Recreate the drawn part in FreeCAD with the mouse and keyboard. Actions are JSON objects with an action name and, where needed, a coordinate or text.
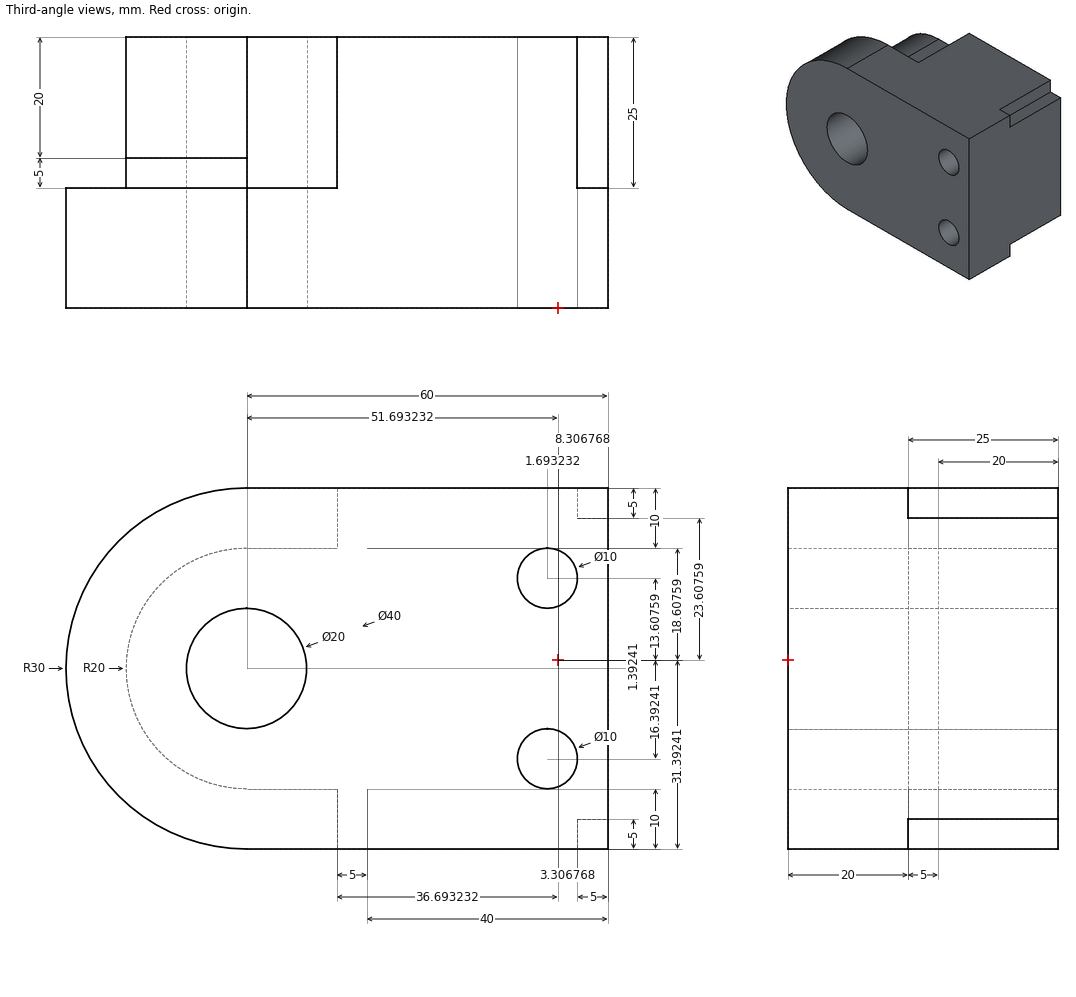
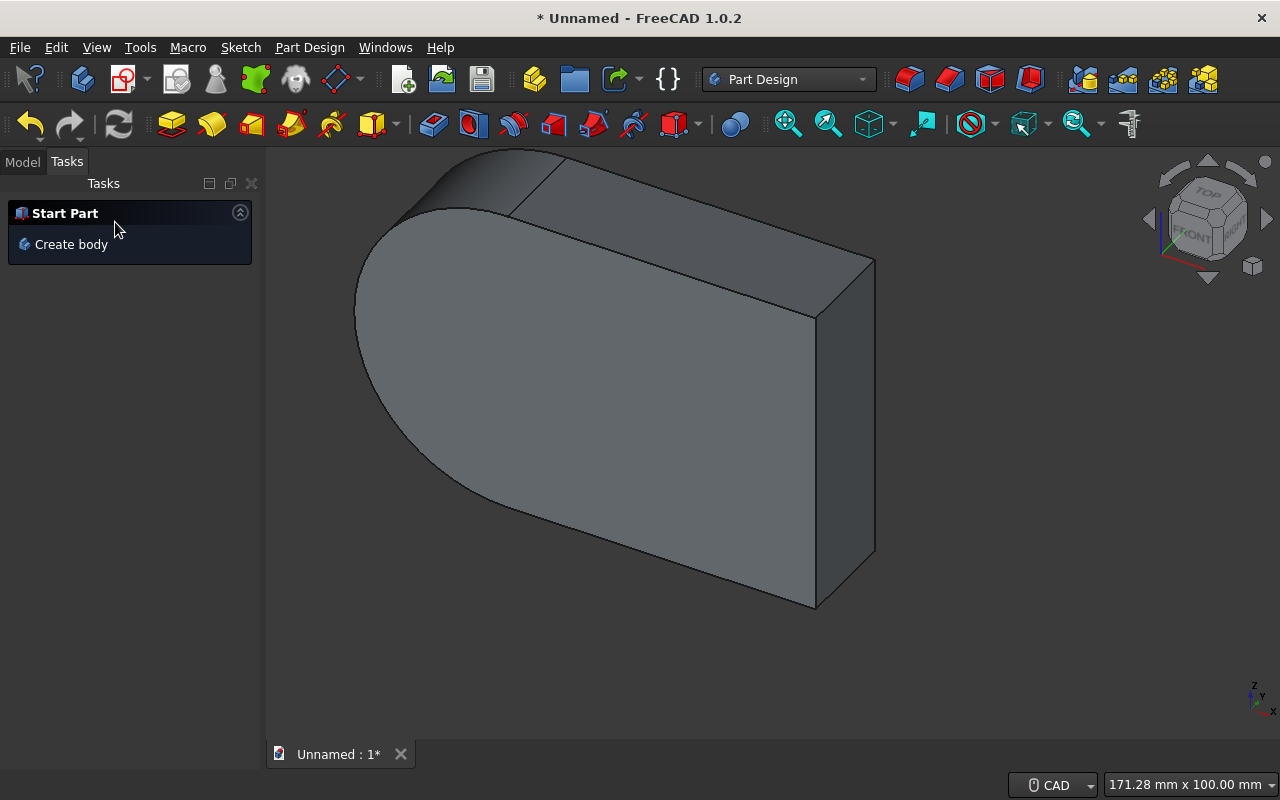
{"action": "key", "text": "v f"}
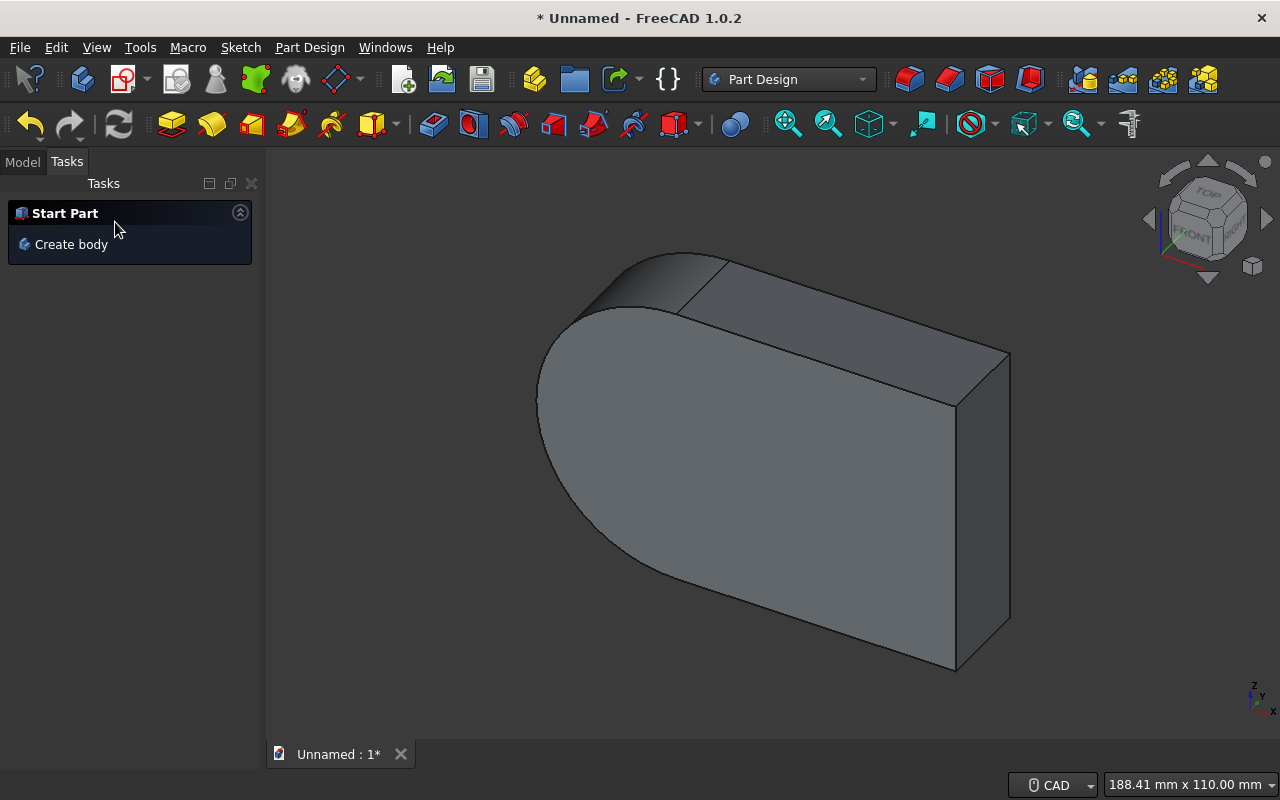
{"action": "key", "text": "4"}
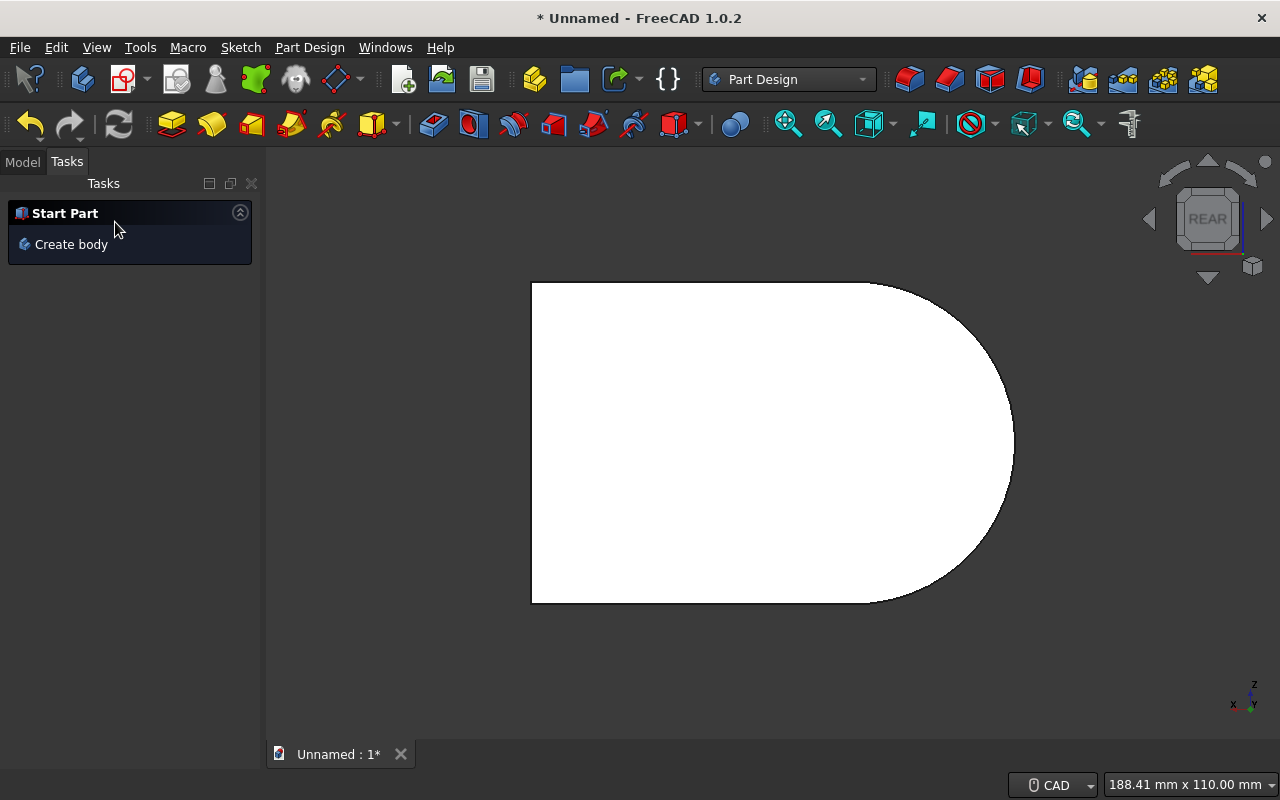
{"action": "left_click", "coordinate": [704, 442]}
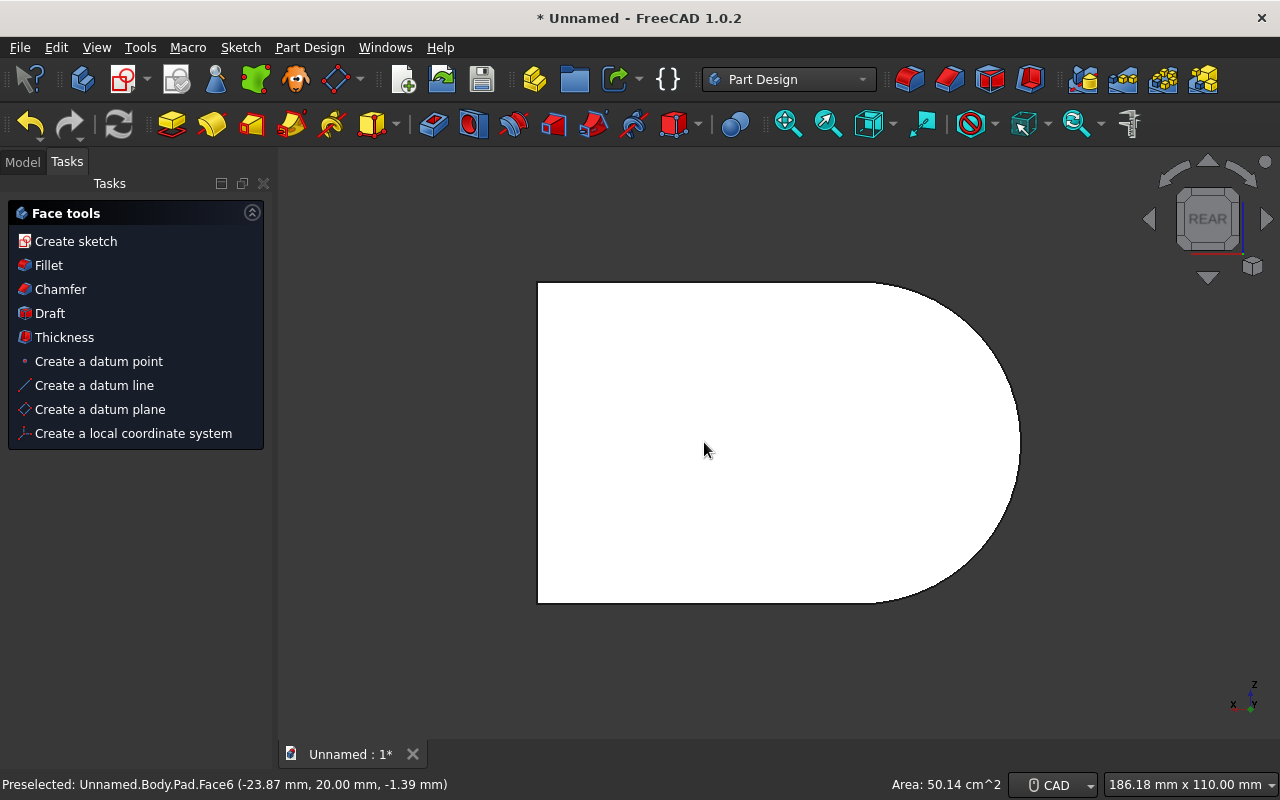
{"action": "left_click", "coordinate": [124, 80]}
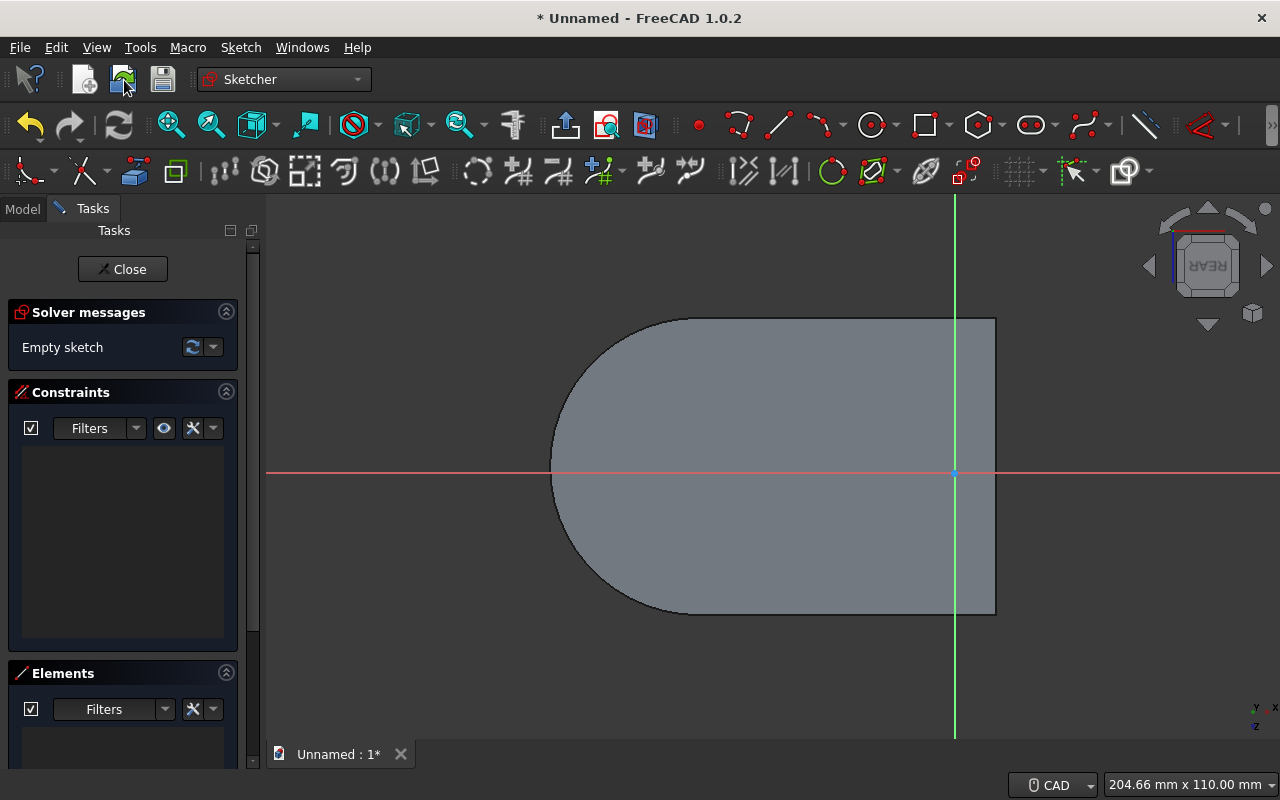
{"action": "scroll", "coordinate": [925, 467], "scroll_direction": "up", "scroll_amount": 2}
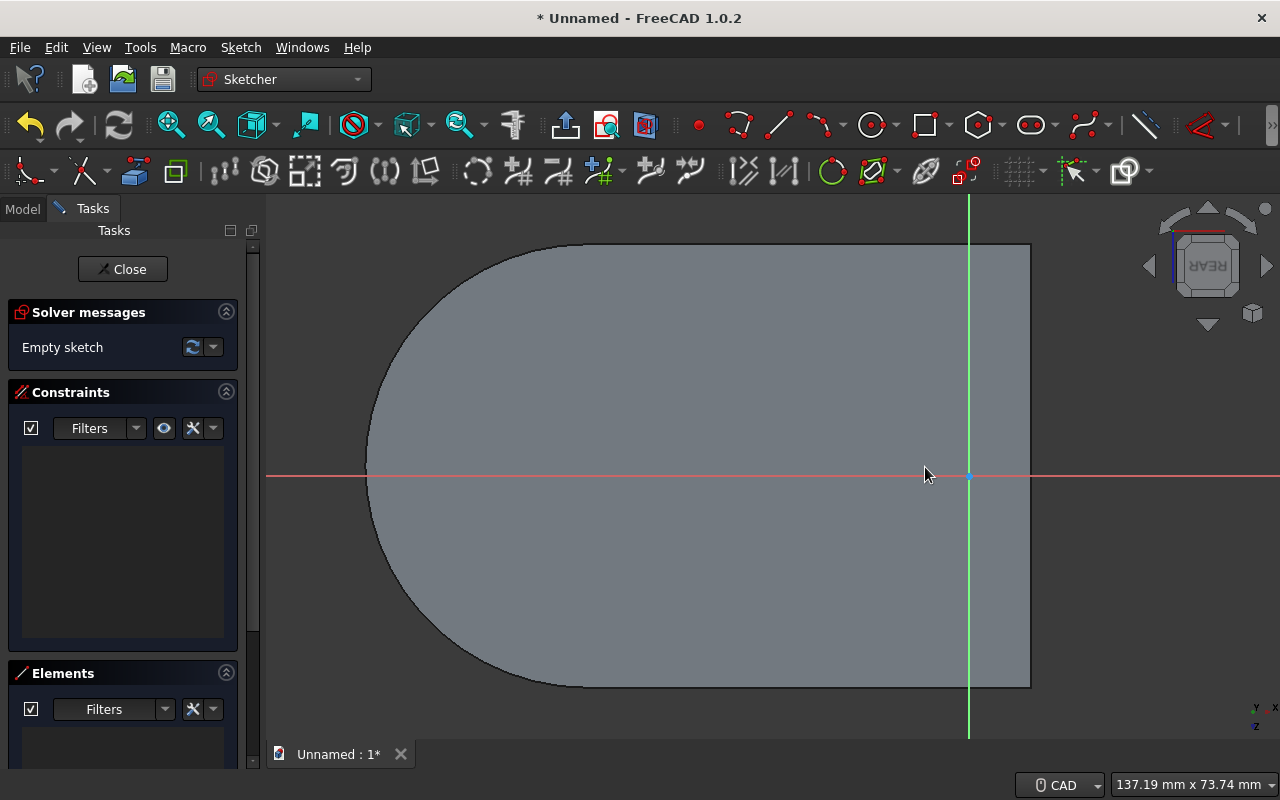
{"action": "key", "text": "g c"}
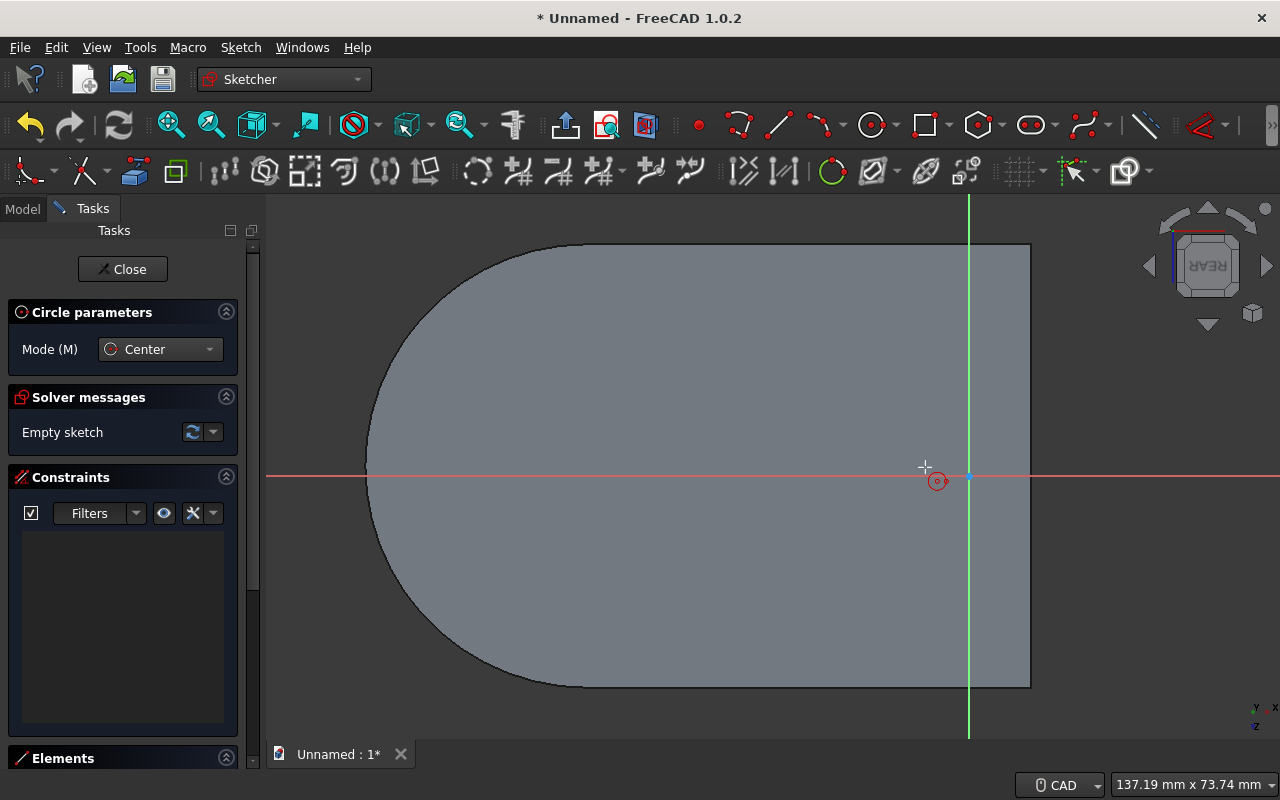
{"action": "scroll", "coordinate": [587, 466], "scroll_direction": "up", "scroll_amount": 3}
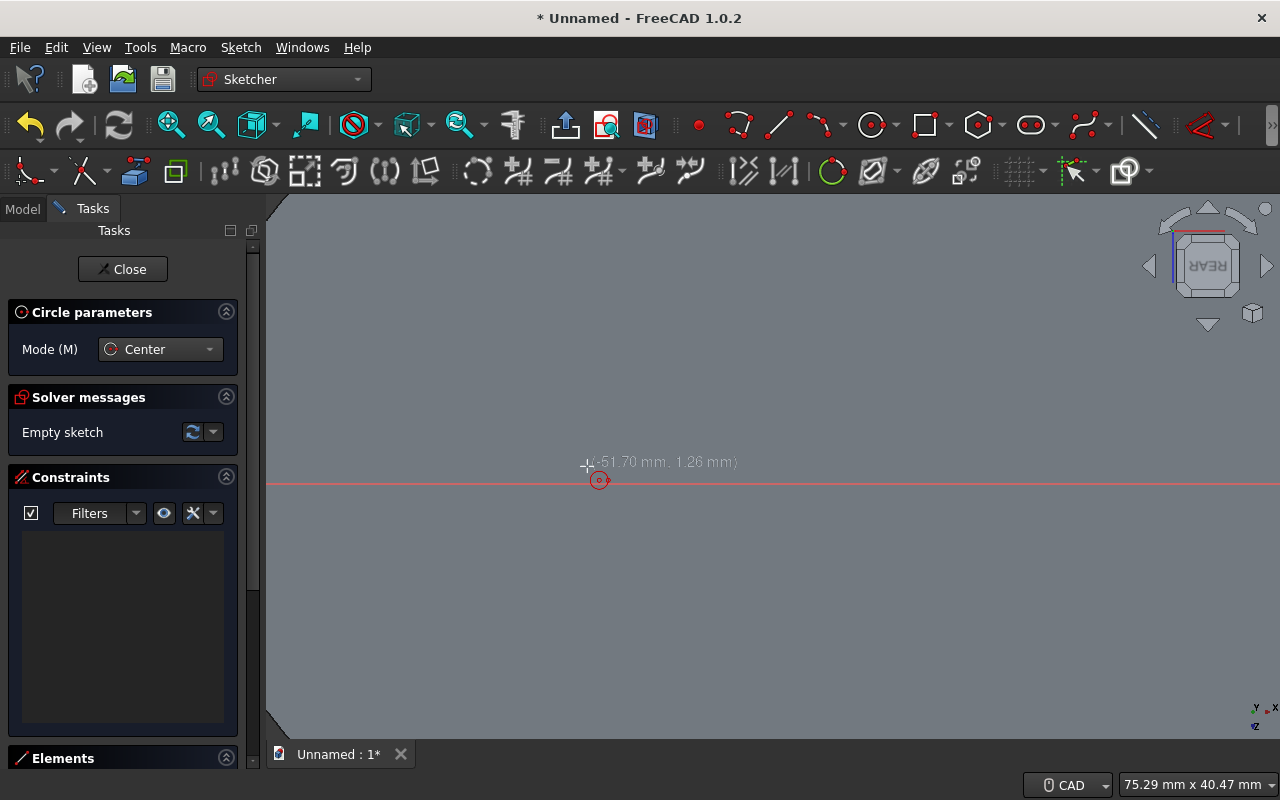
{"action": "left_click", "coordinate": [587, 466]}
{"action": "left_click", "coordinate": [777, 275]}
{"action": "key", "text": "Escape"}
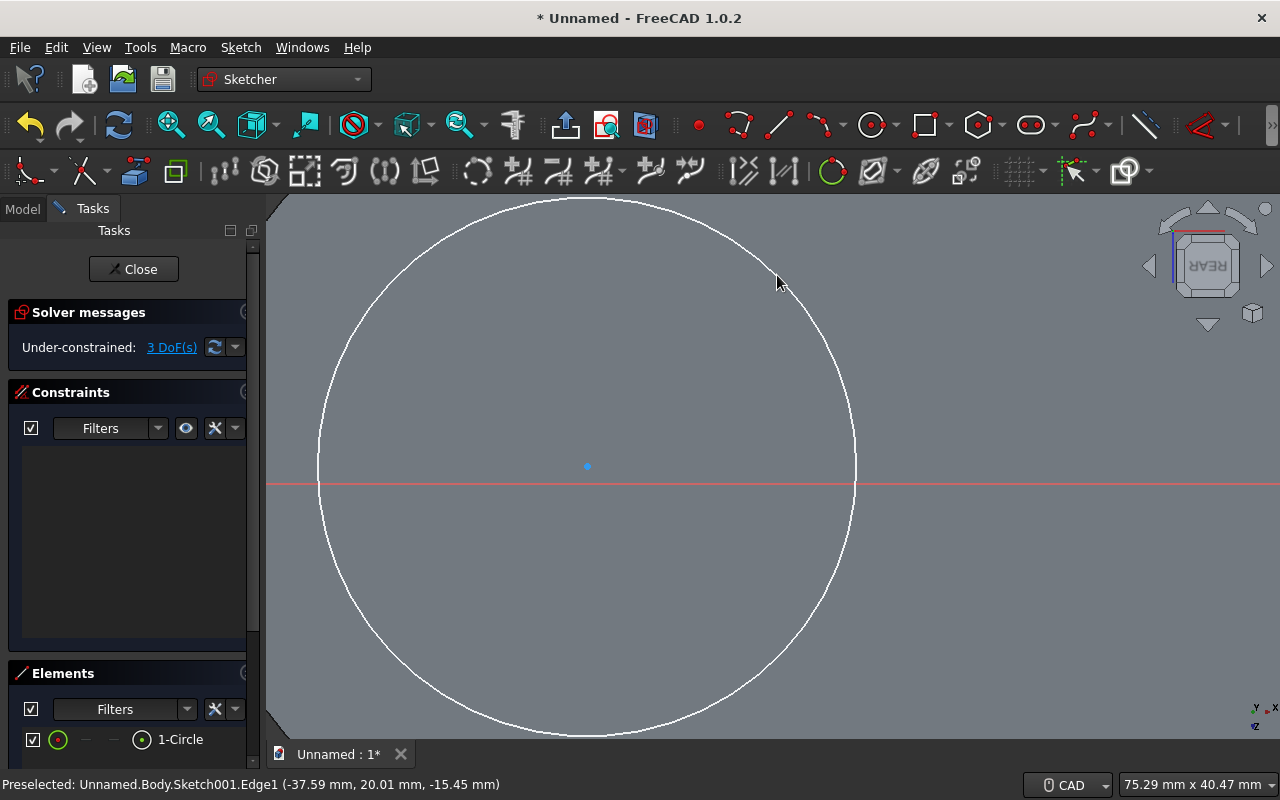
{"action": "key", "text": "d"}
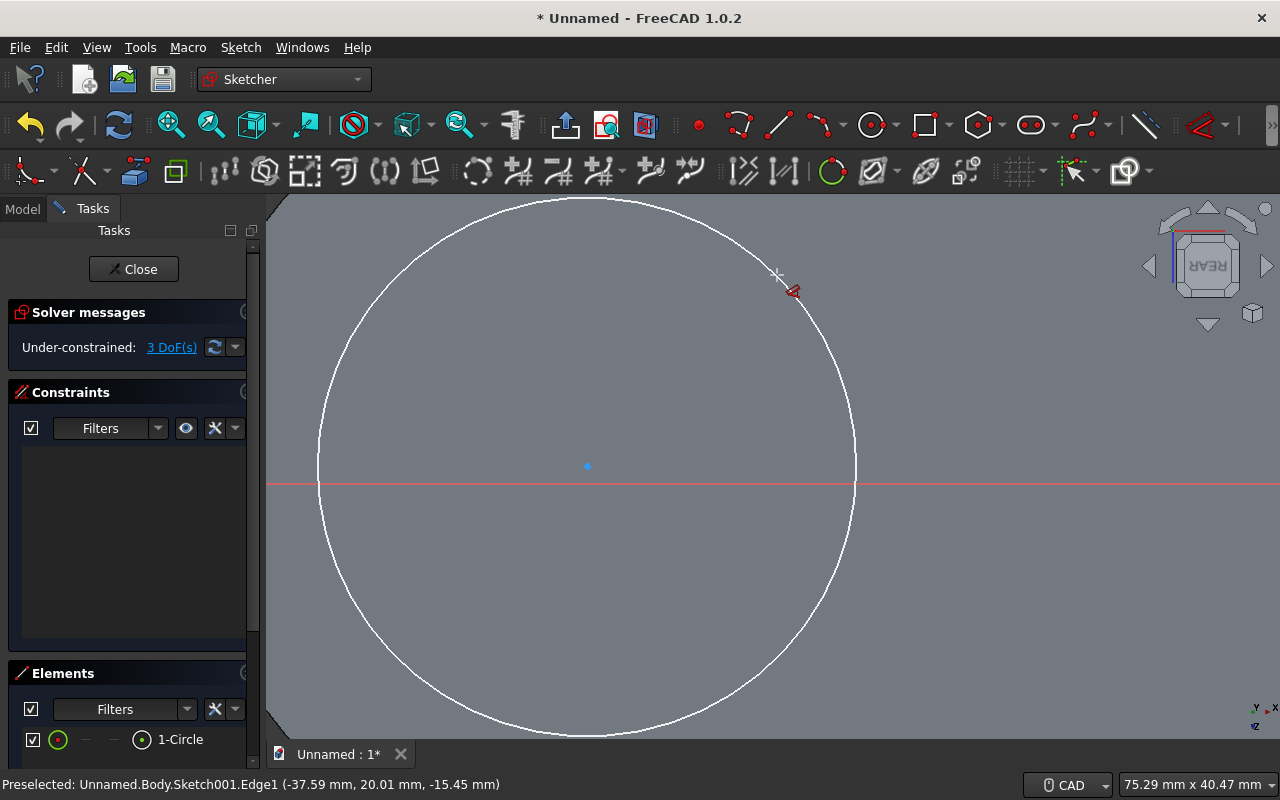
{"action": "left_click", "coordinate": [777, 276]}
{"action": "left_click", "coordinate": [800, 253]}